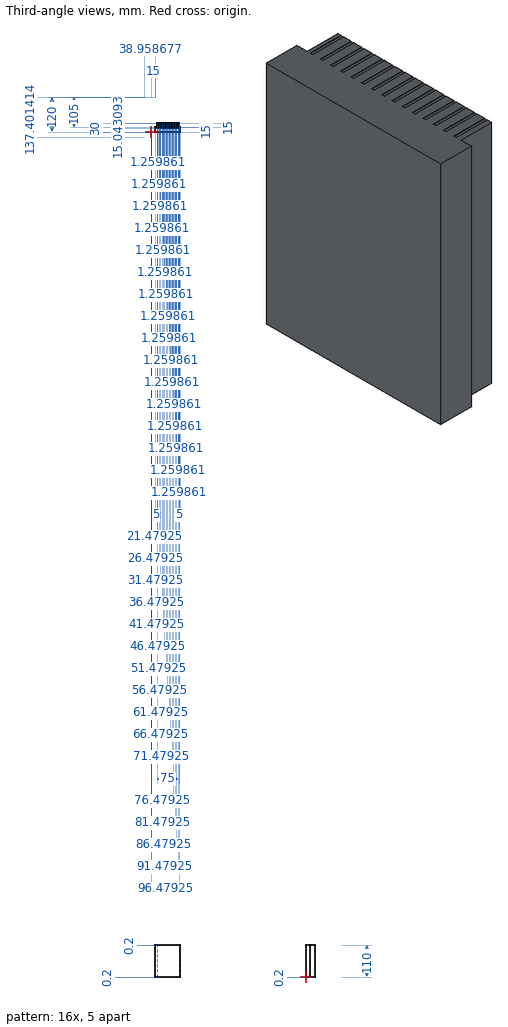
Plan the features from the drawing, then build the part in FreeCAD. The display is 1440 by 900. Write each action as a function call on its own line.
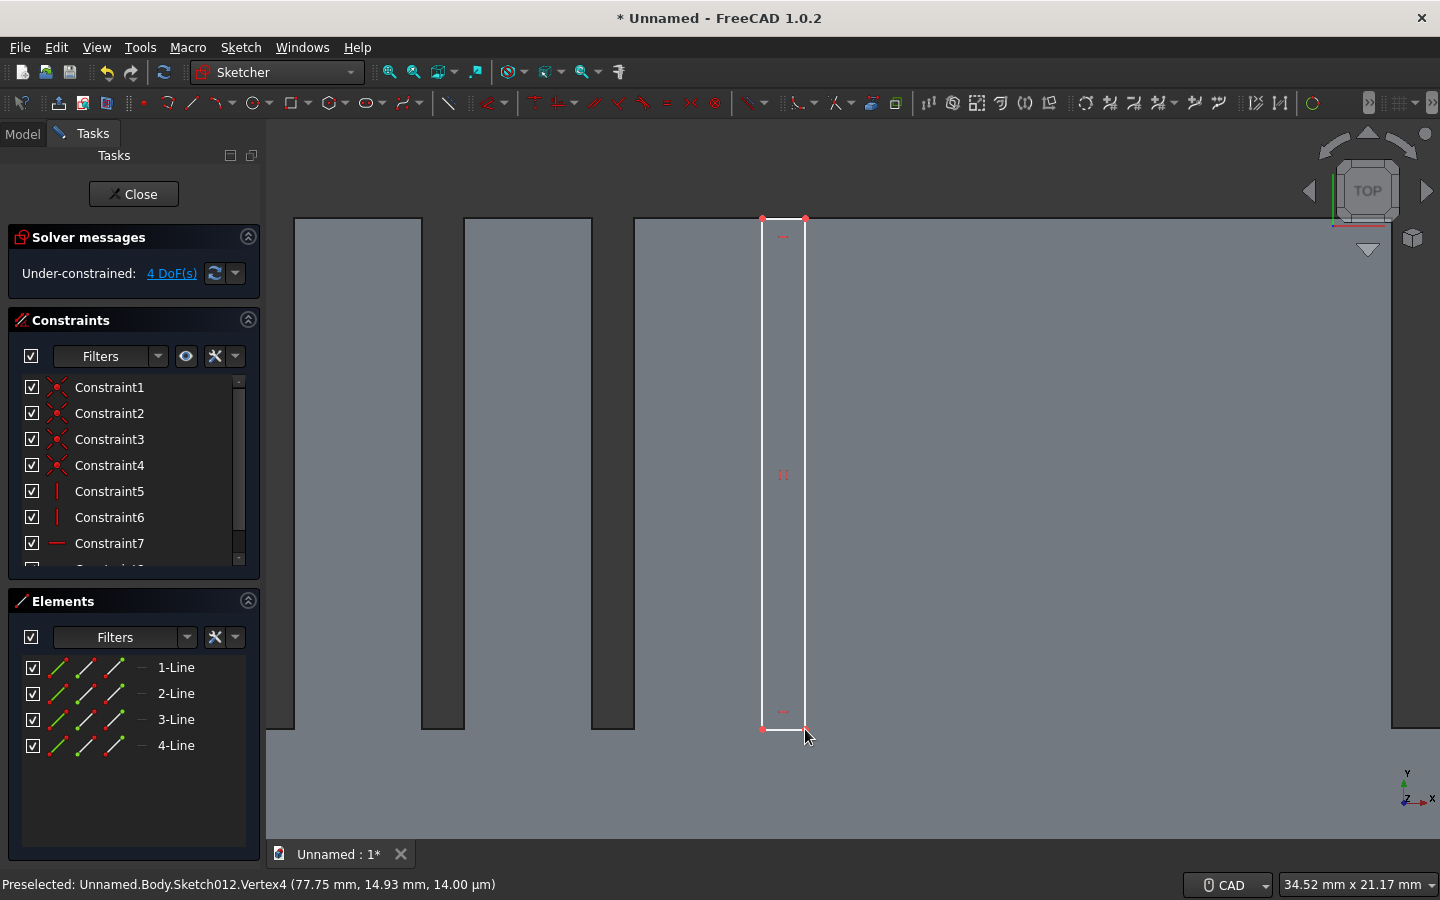
key(d)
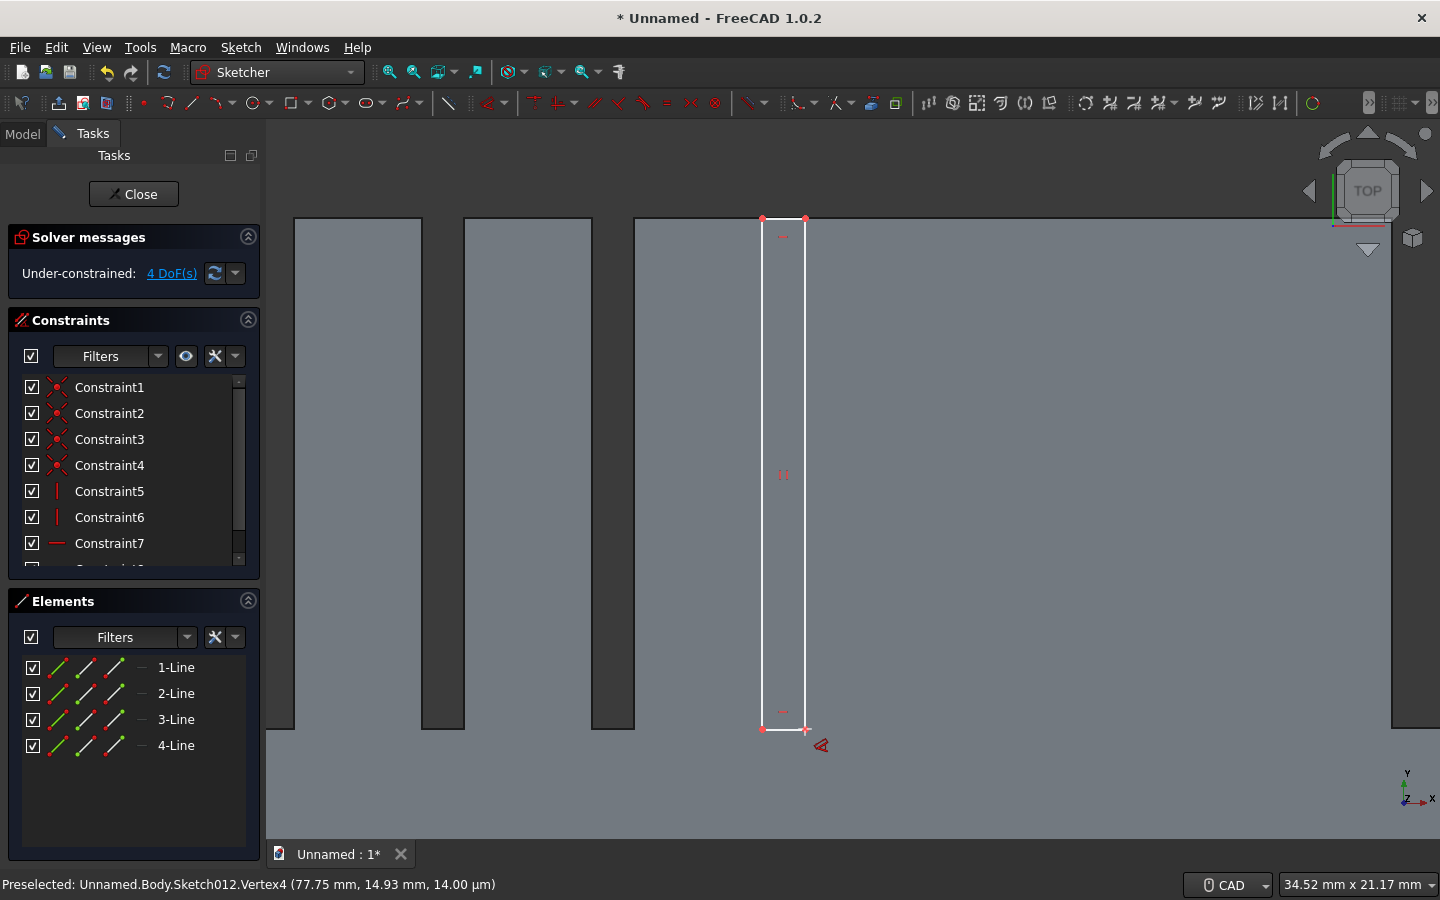
click(762, 219)
click(820, 515)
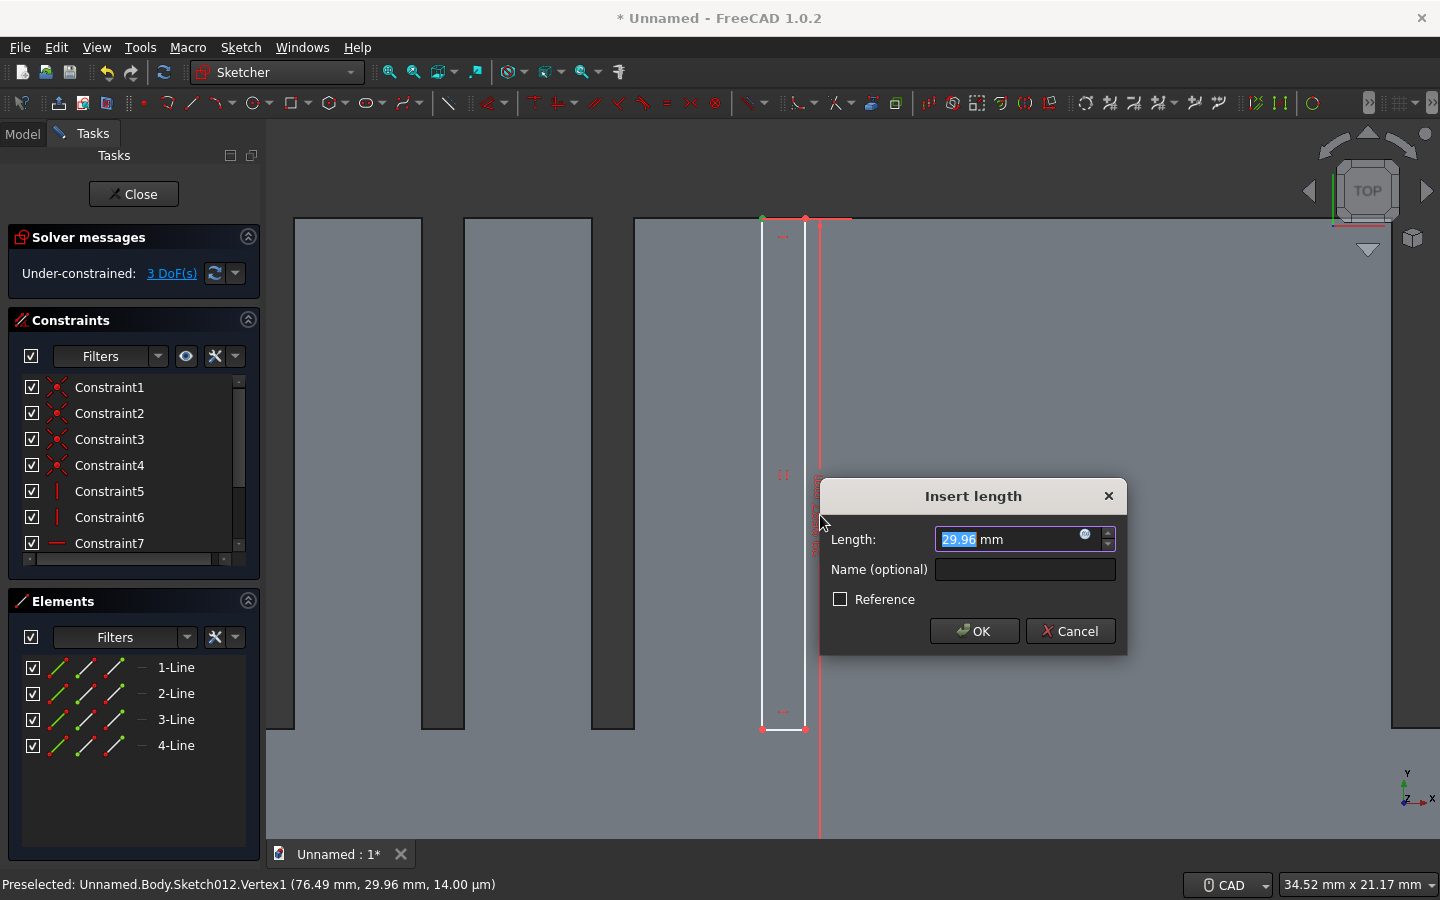
text(30)
key(Return)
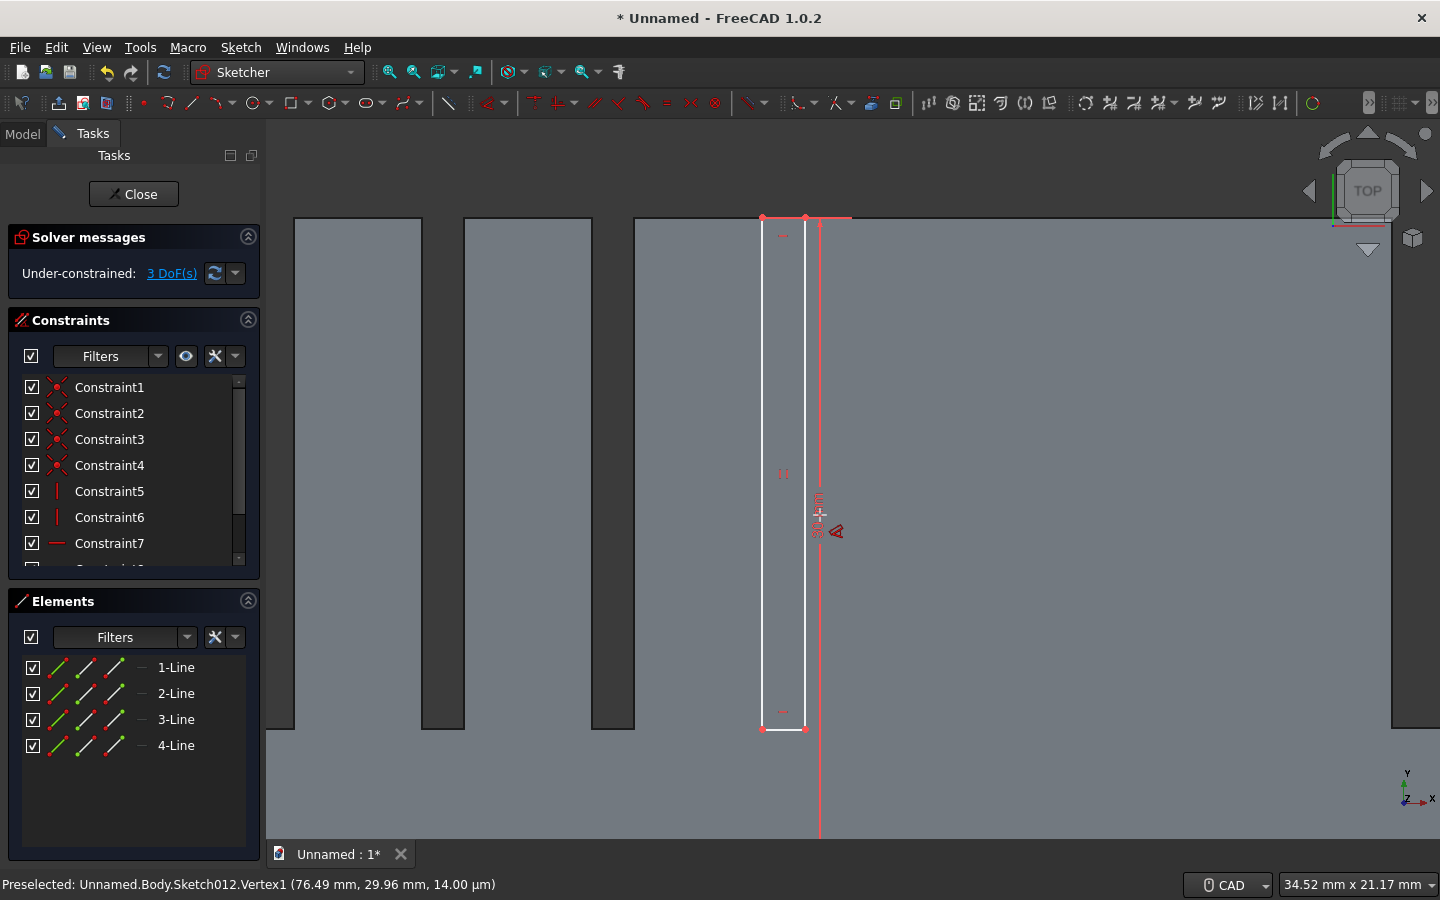
click(775, 730)
click(784, 764)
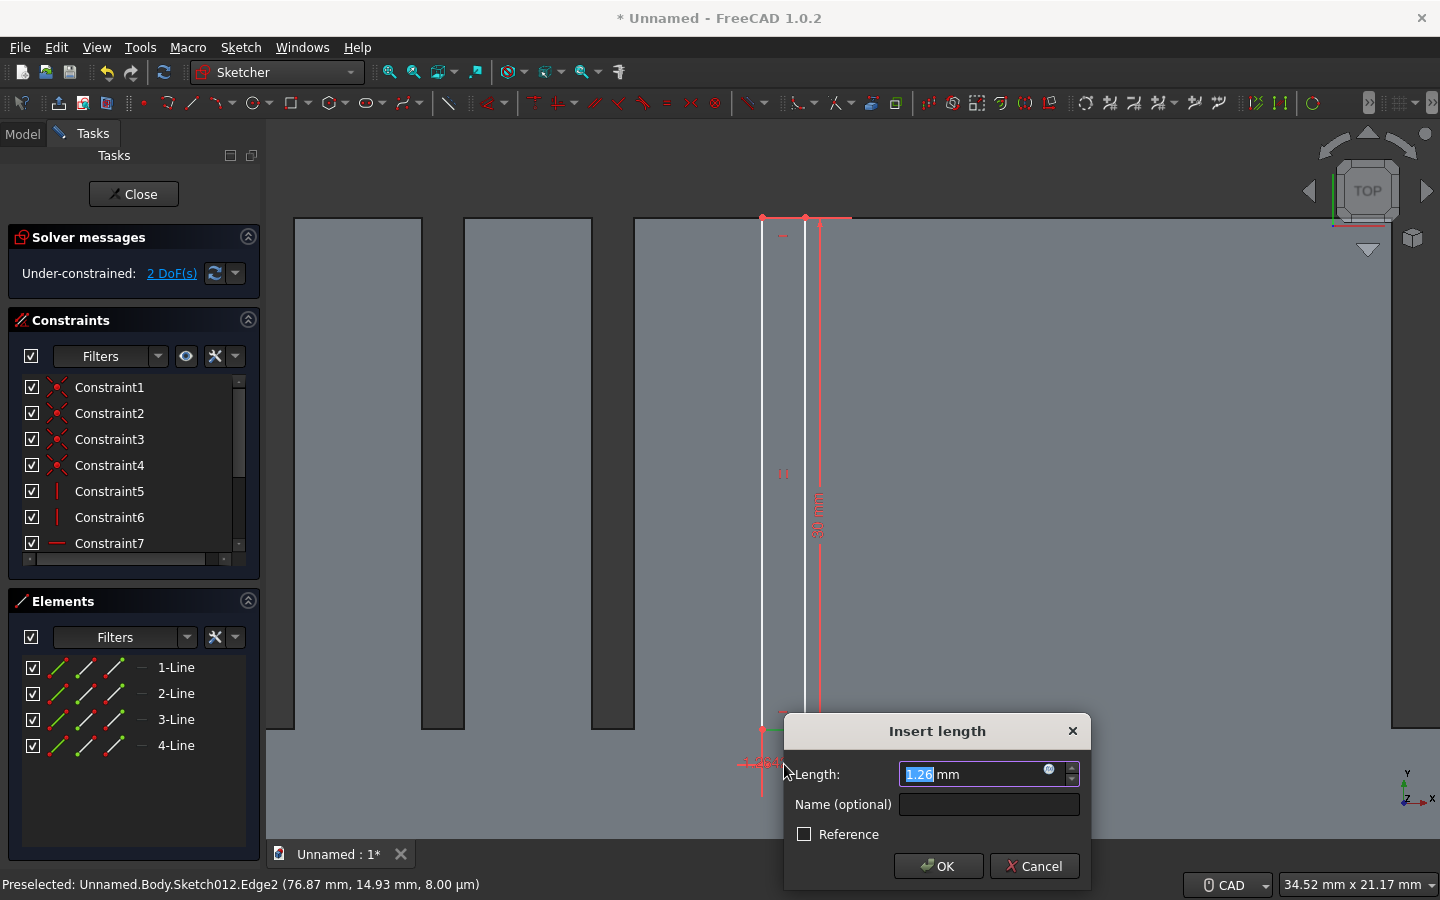
text(1.259861)
key(Return)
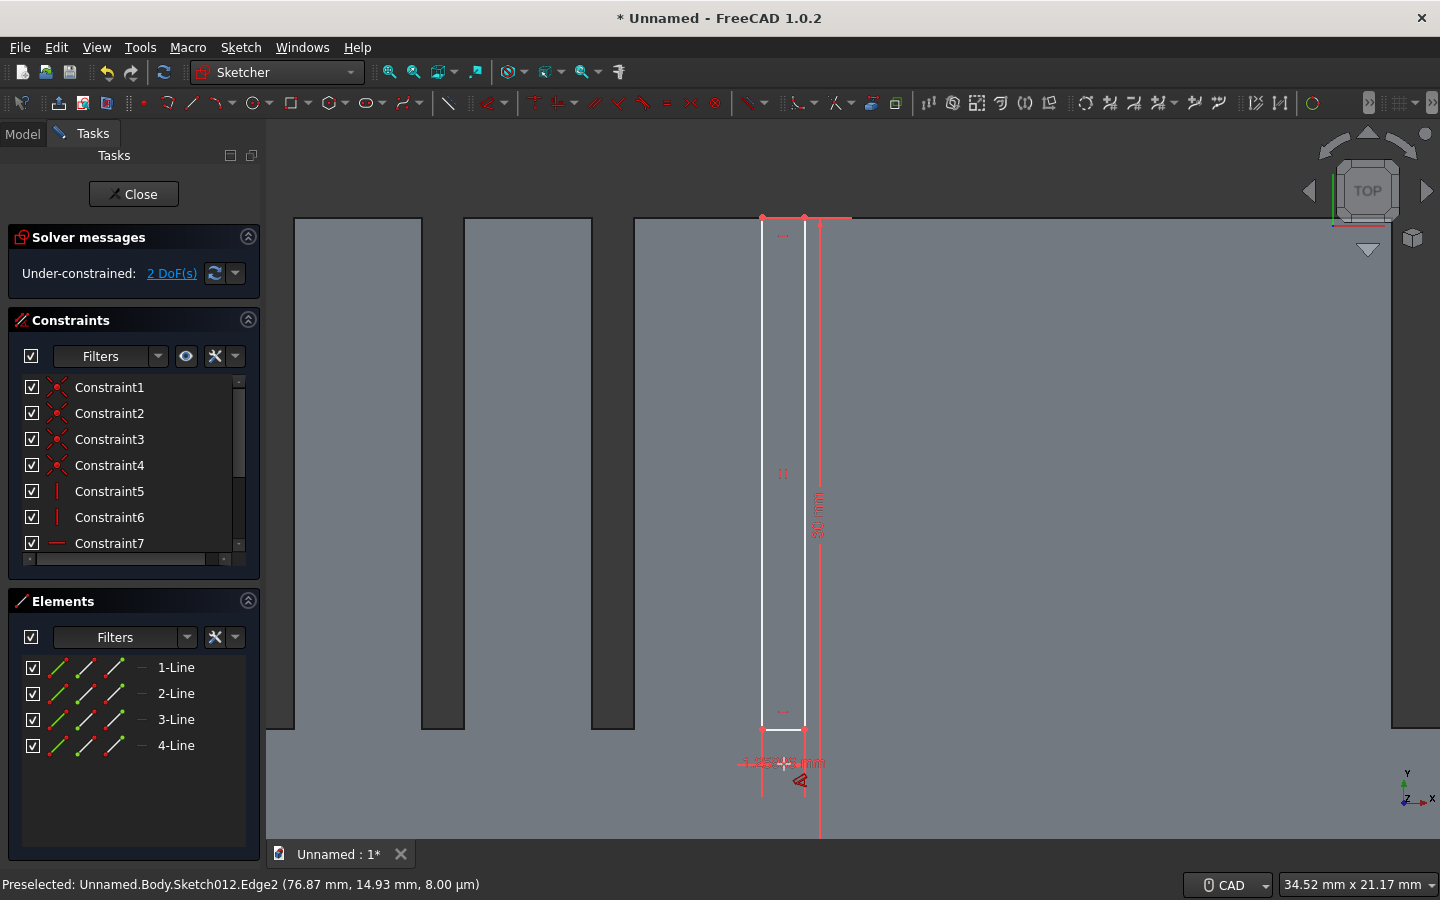
click(762, 371)
click(728, 474)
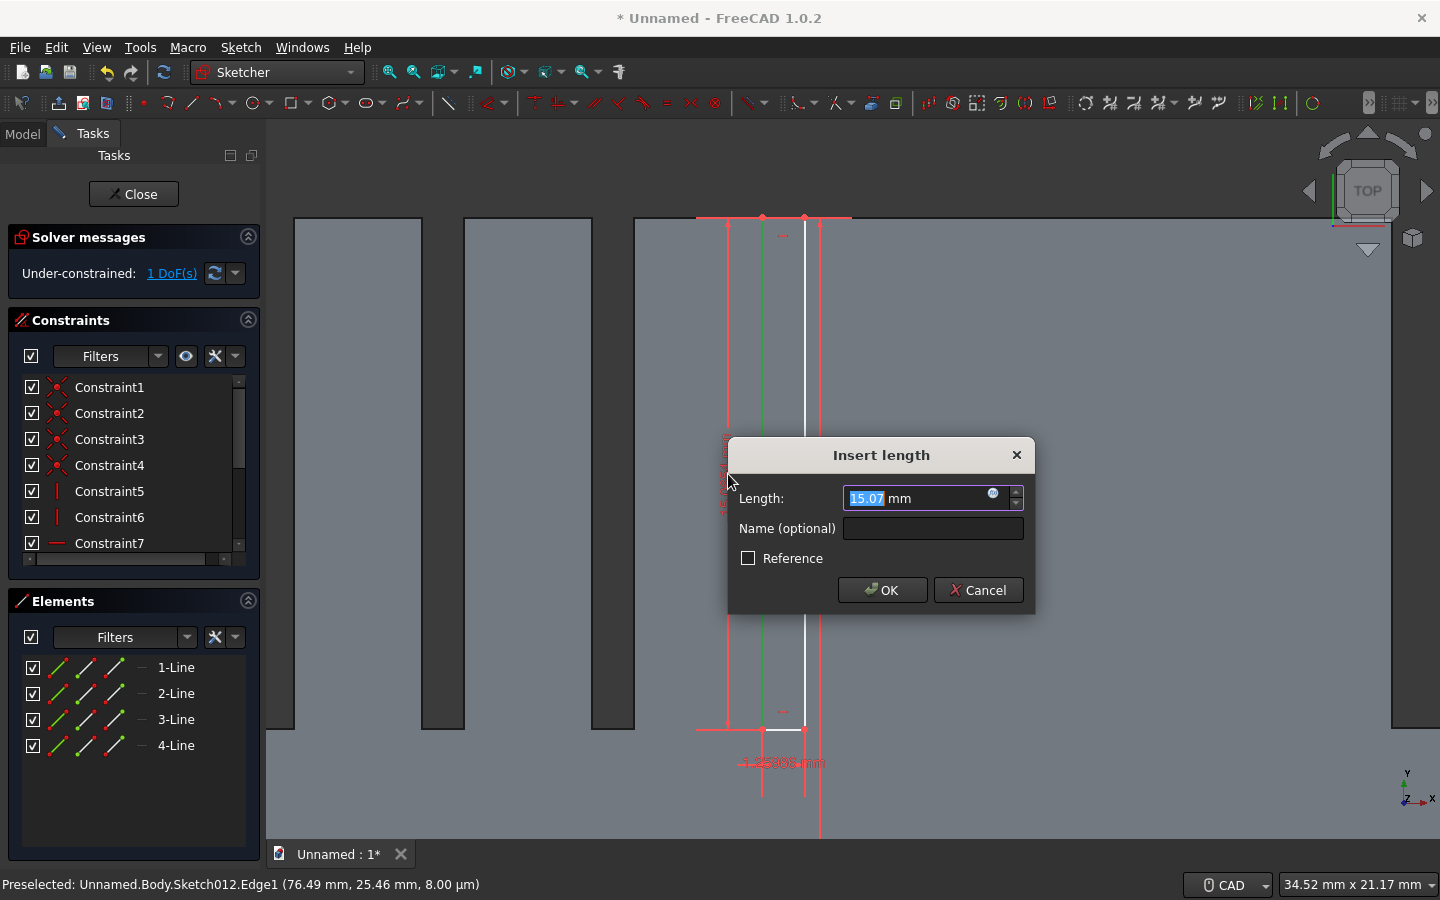
text(15.043093)
key(Return)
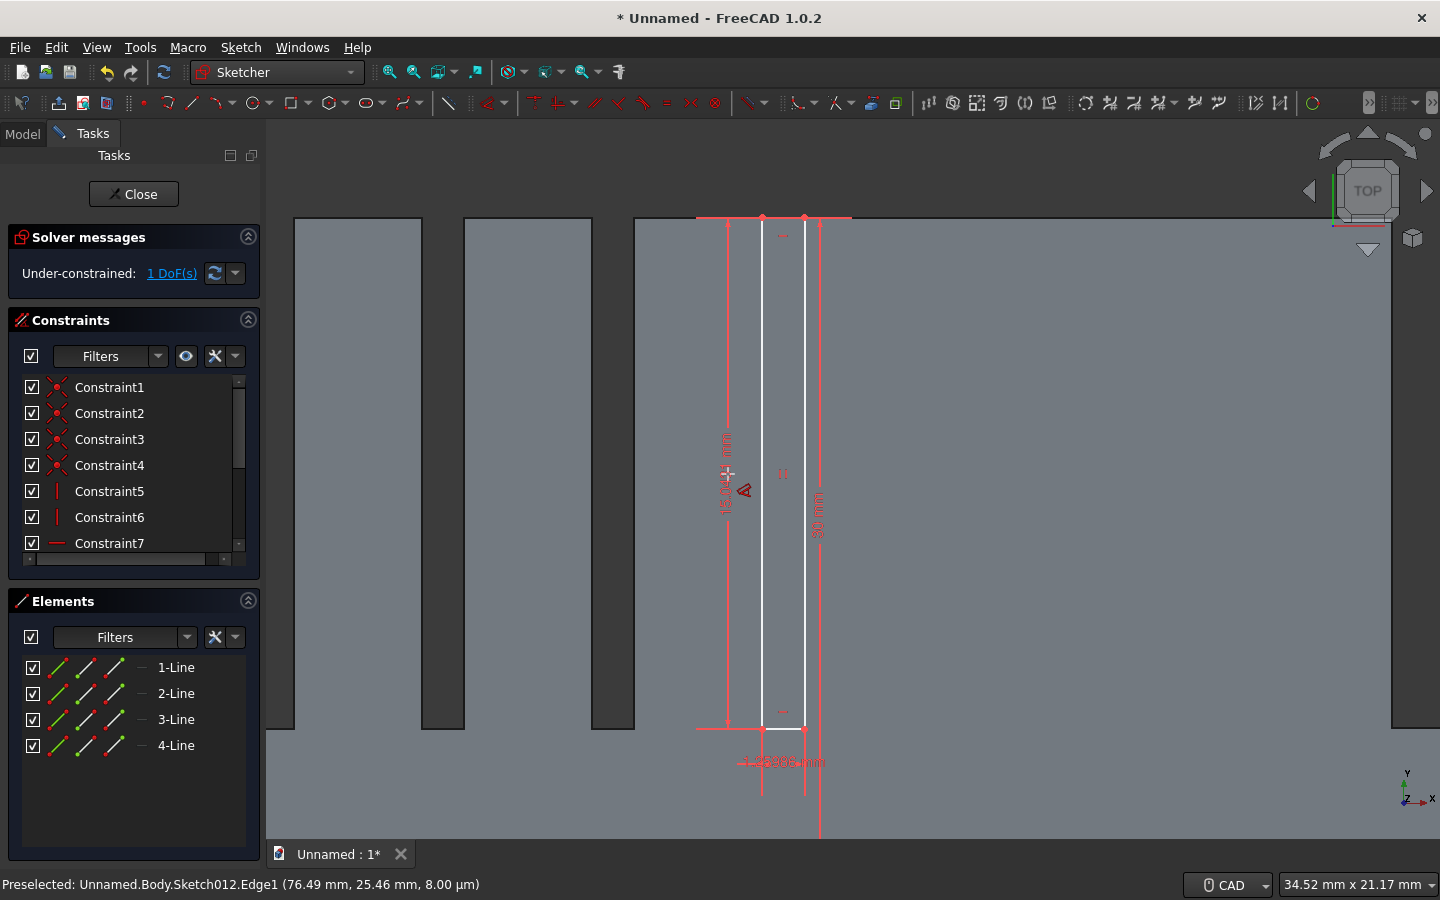
click(762, 218)
click(528, 184)